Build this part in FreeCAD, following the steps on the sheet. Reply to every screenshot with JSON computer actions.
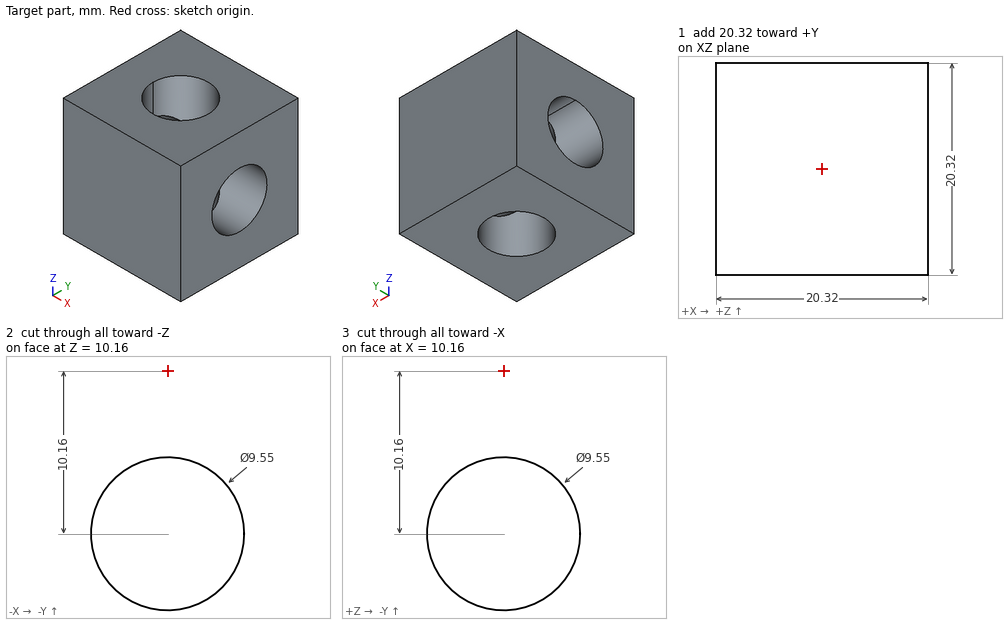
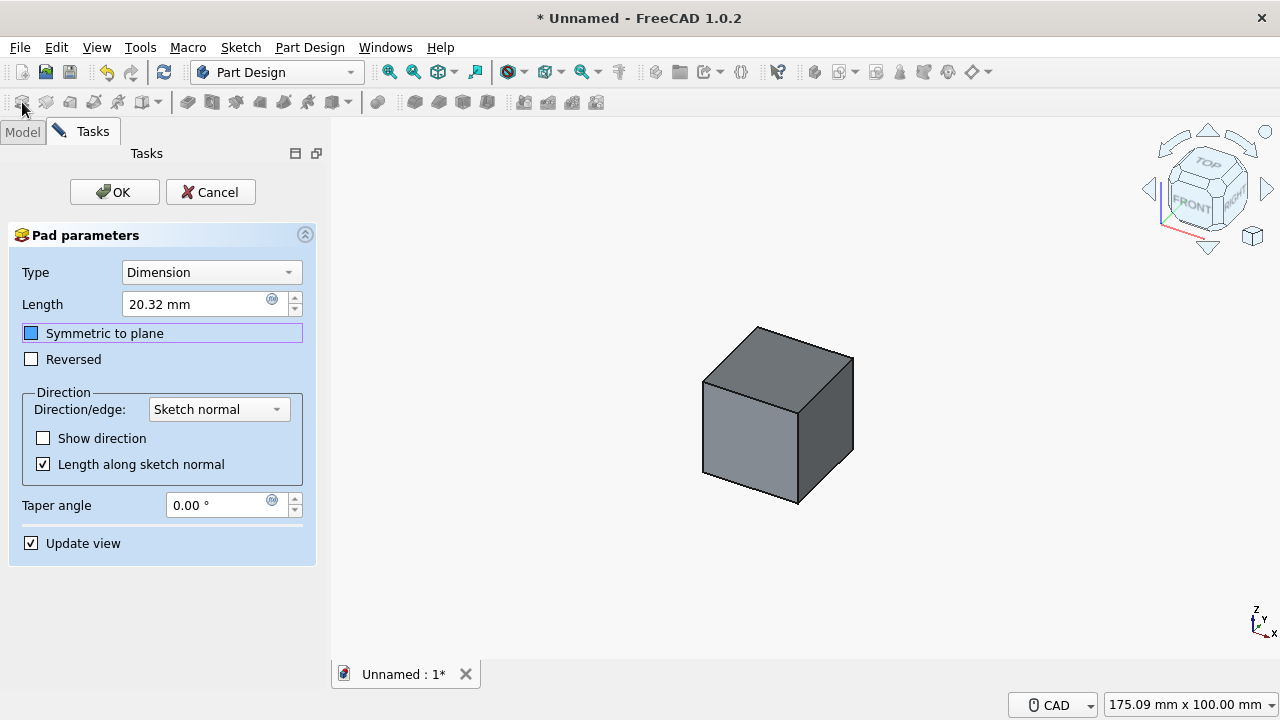
{"action": "left_click", "coordinate": [30, 359]}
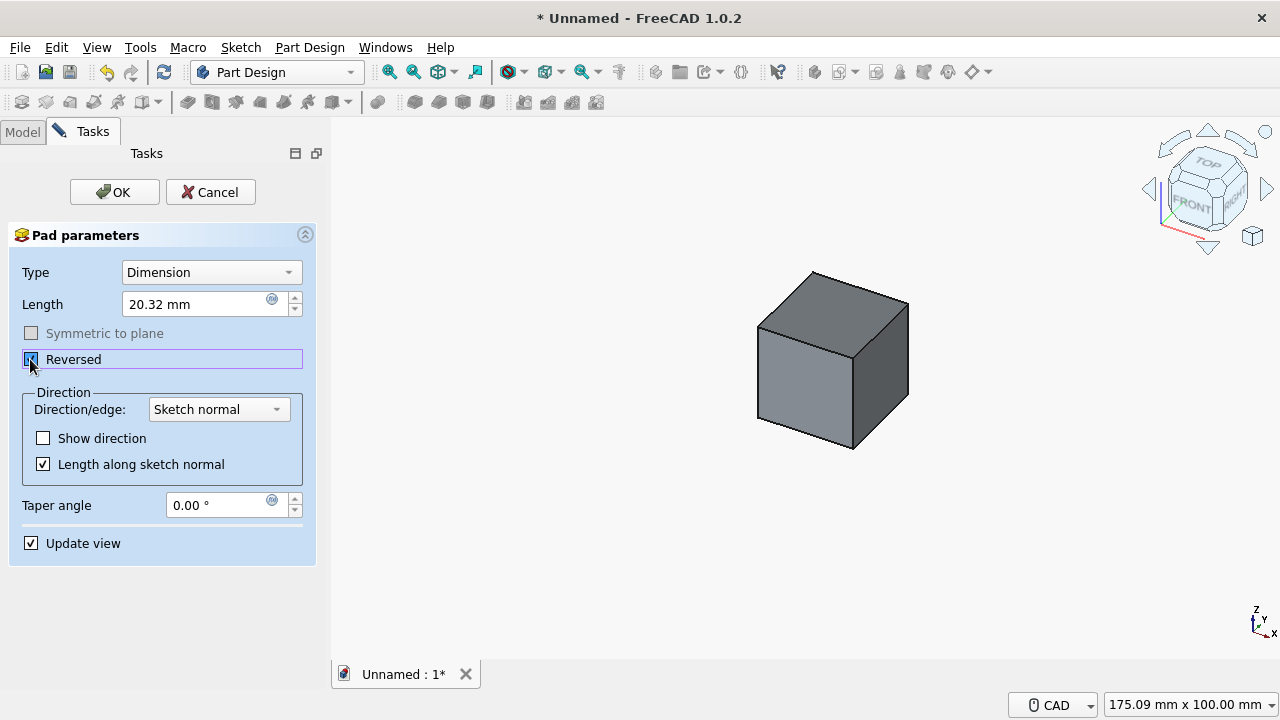
{"action": "left_click", "coordinate": [115, 192]}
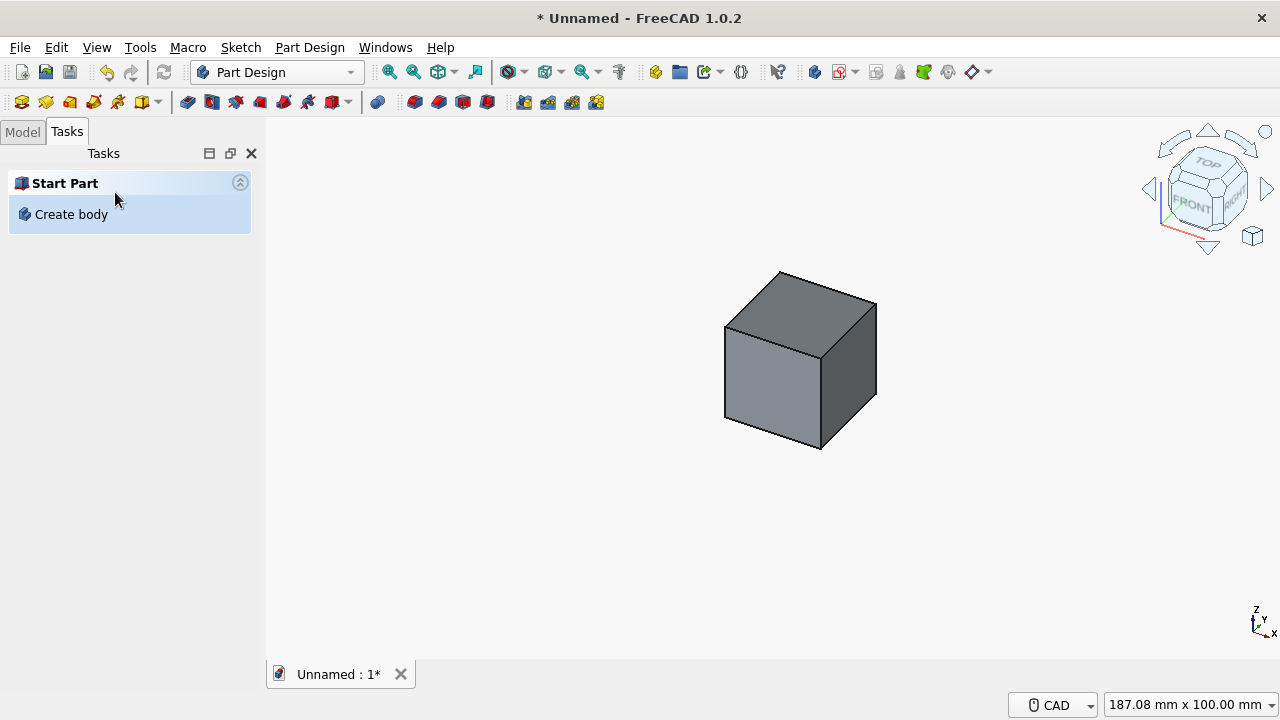
{"action": "key", "text": "v f"}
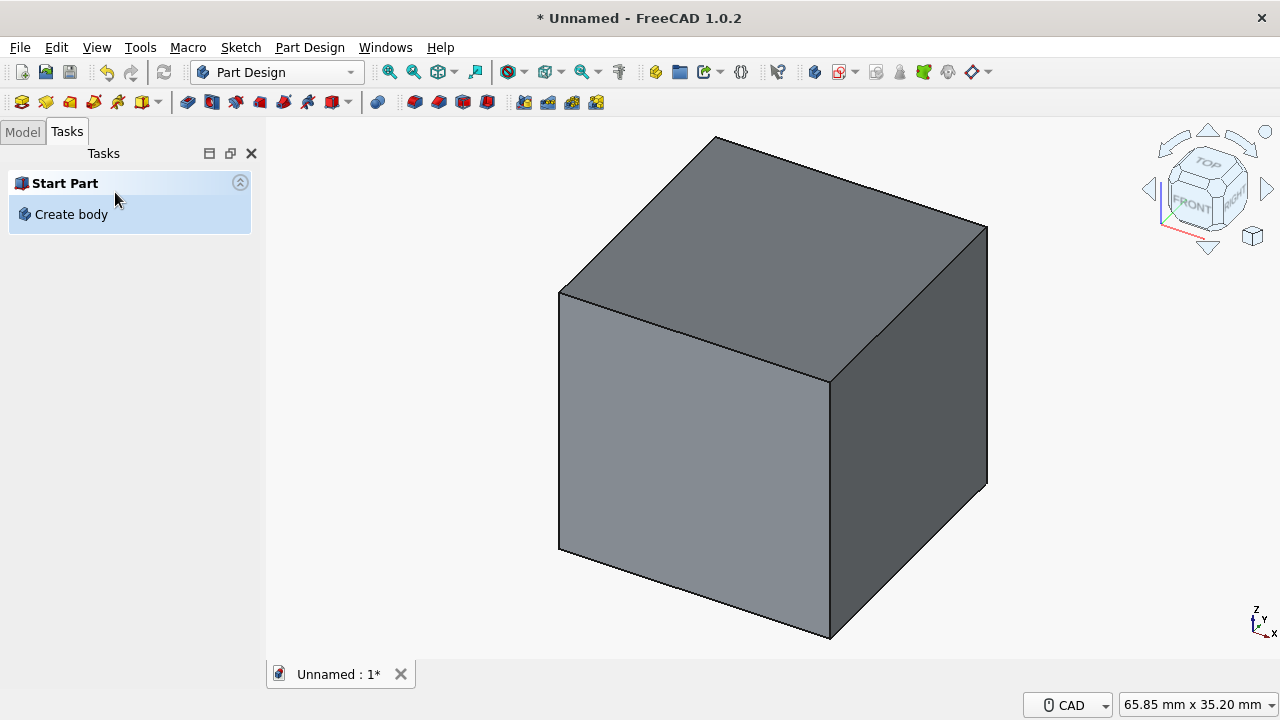
{"action": "left_click", "coordinate": [773, 259]}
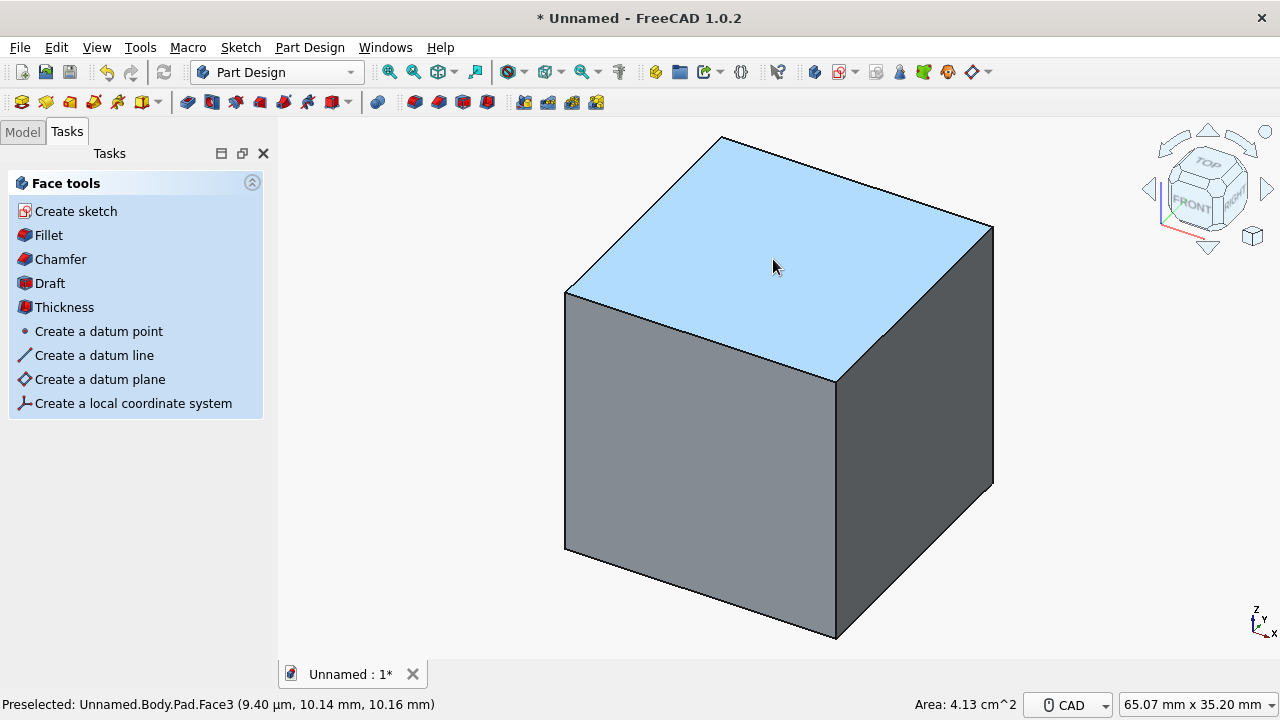
{"action": "left_click", "coordinate": [840, 72]}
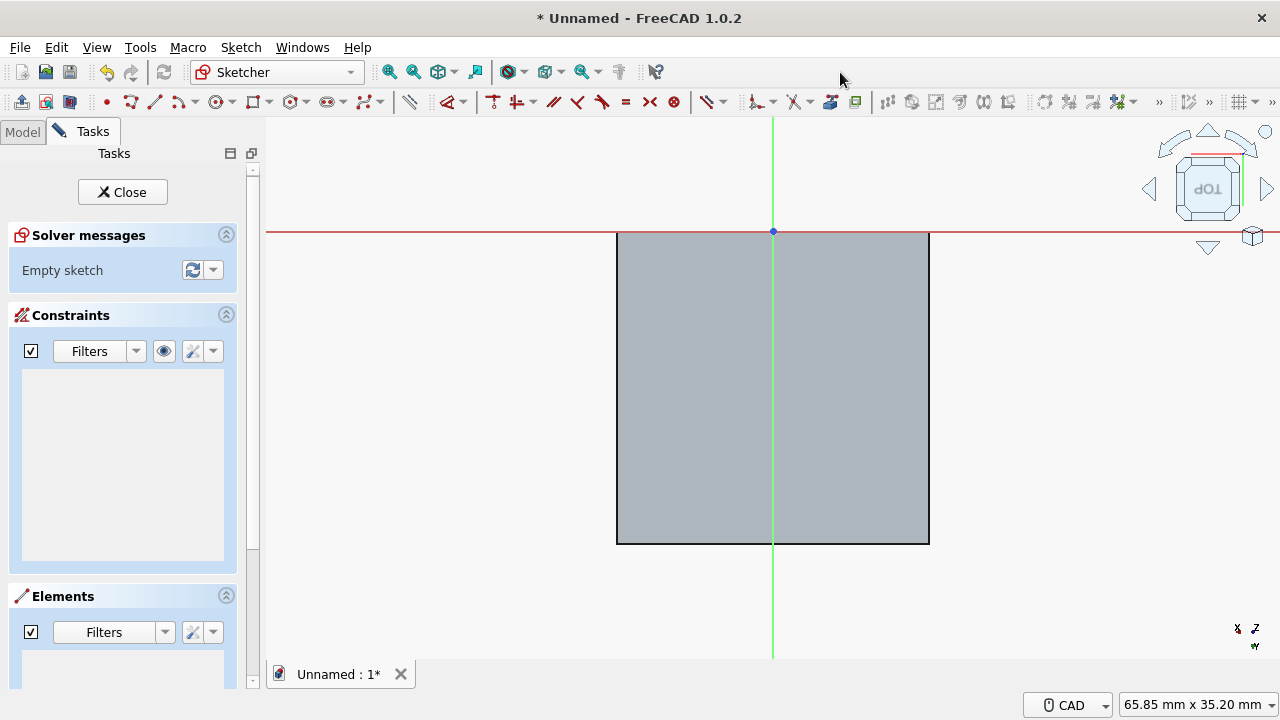
{"action": "scroll", "coordinate": [912, 262], "scroll_direction": "up", "scroll_amount": 2}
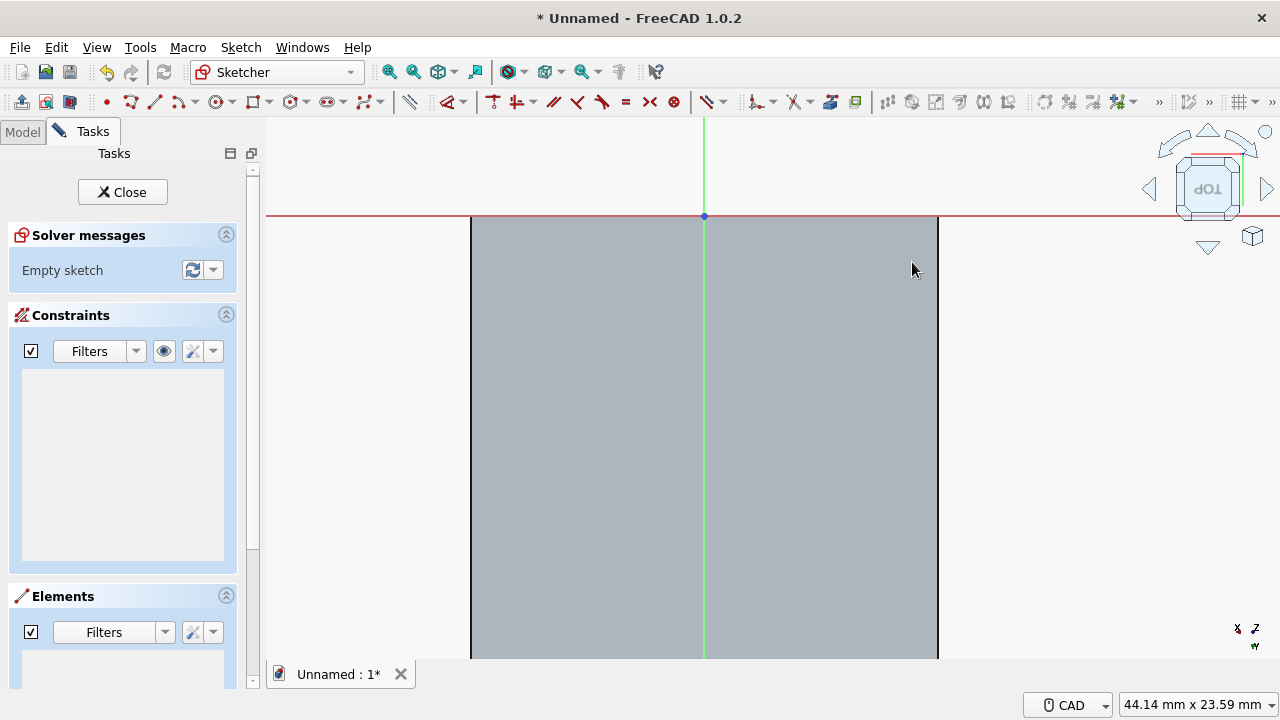
{"action": "key", "text": "g c"}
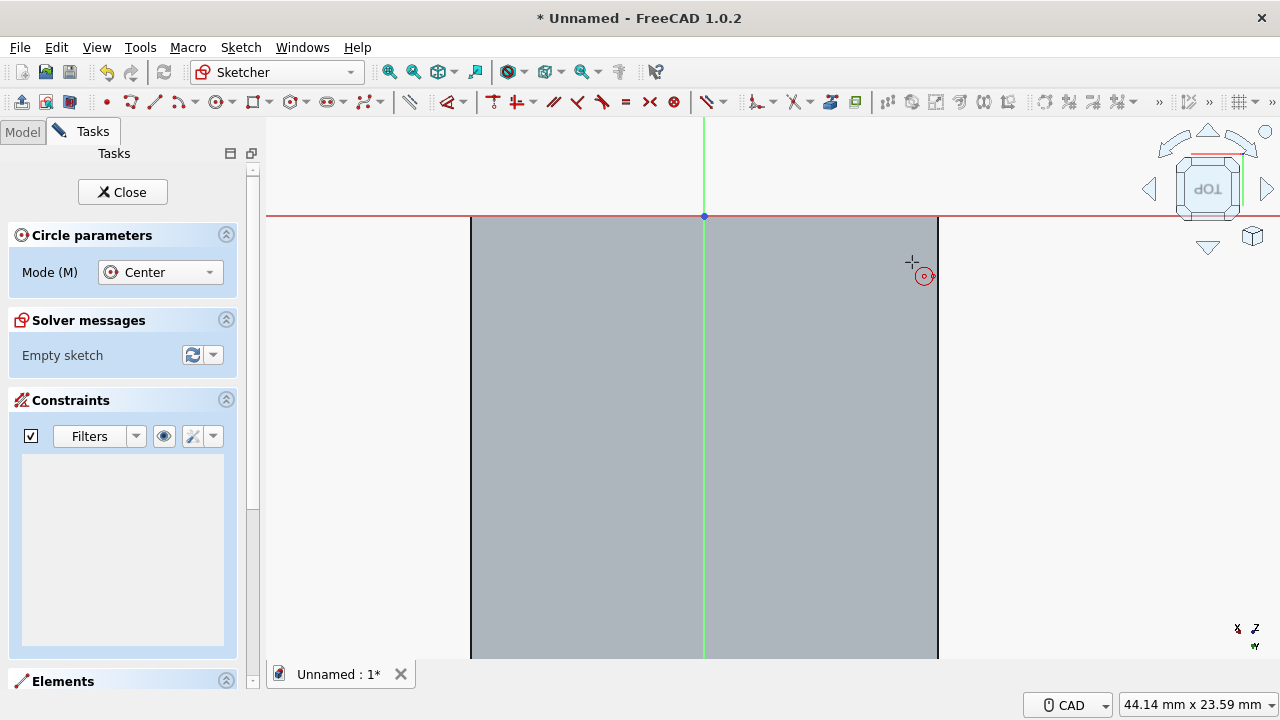
{"action": "left_click", "coordinate": [704, 450]}
{"action": "mouse_move", "coordinate": [782, 372]}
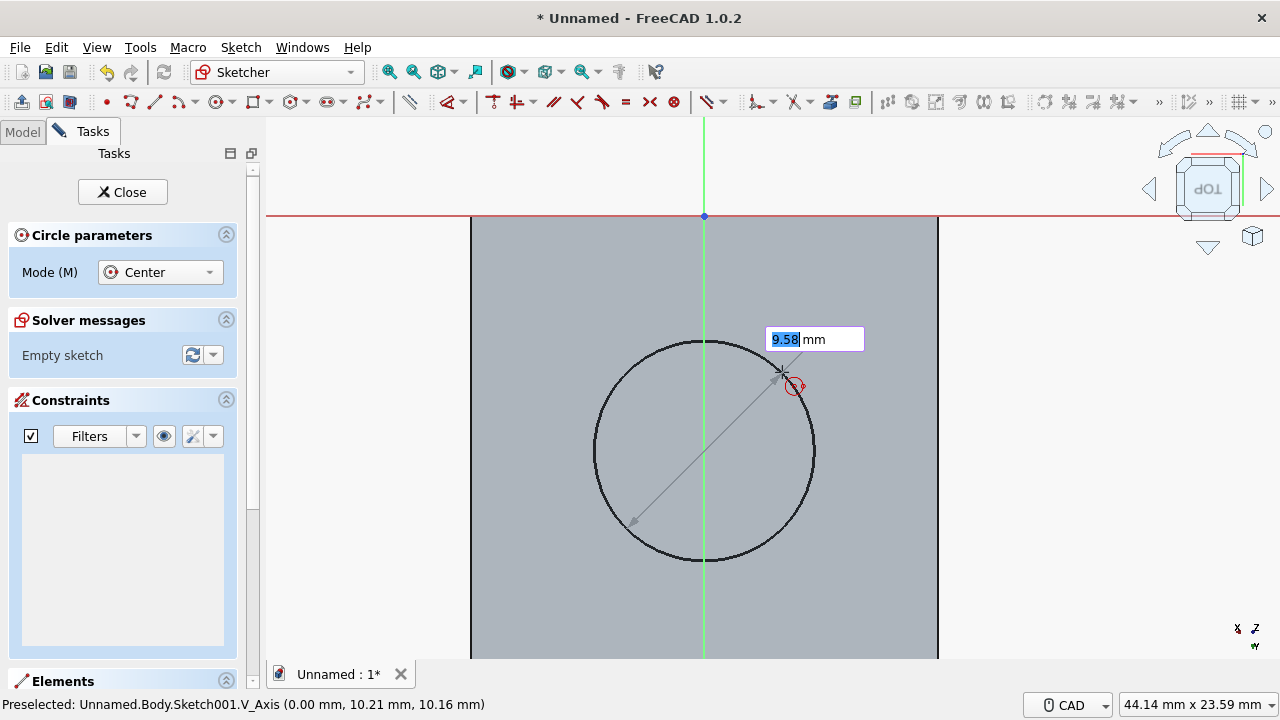
{"action": "type", "text": "9.55"}
{"action": "key", "text": "Return"}
{"action": "key", "text": "Escape"}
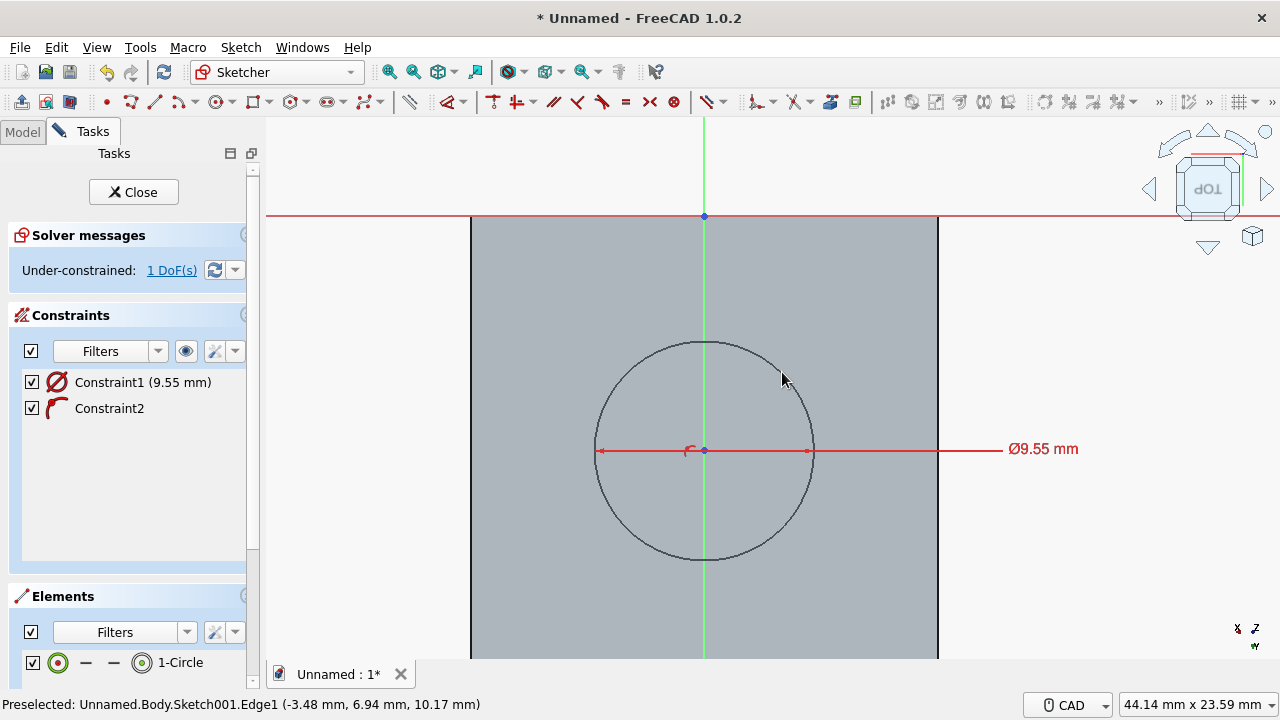
{"action": "left_click", "coordinate": [704, 451]}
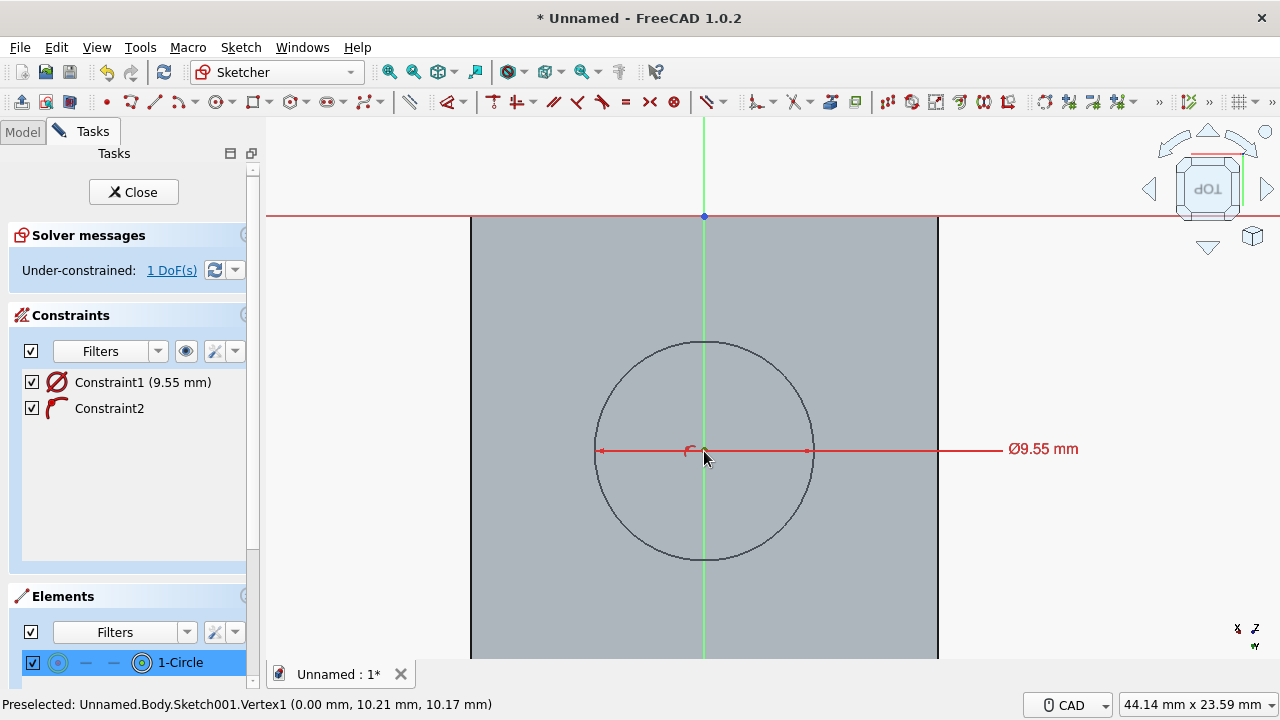
{"action": "left_click", "coordinate": [466, 102]}